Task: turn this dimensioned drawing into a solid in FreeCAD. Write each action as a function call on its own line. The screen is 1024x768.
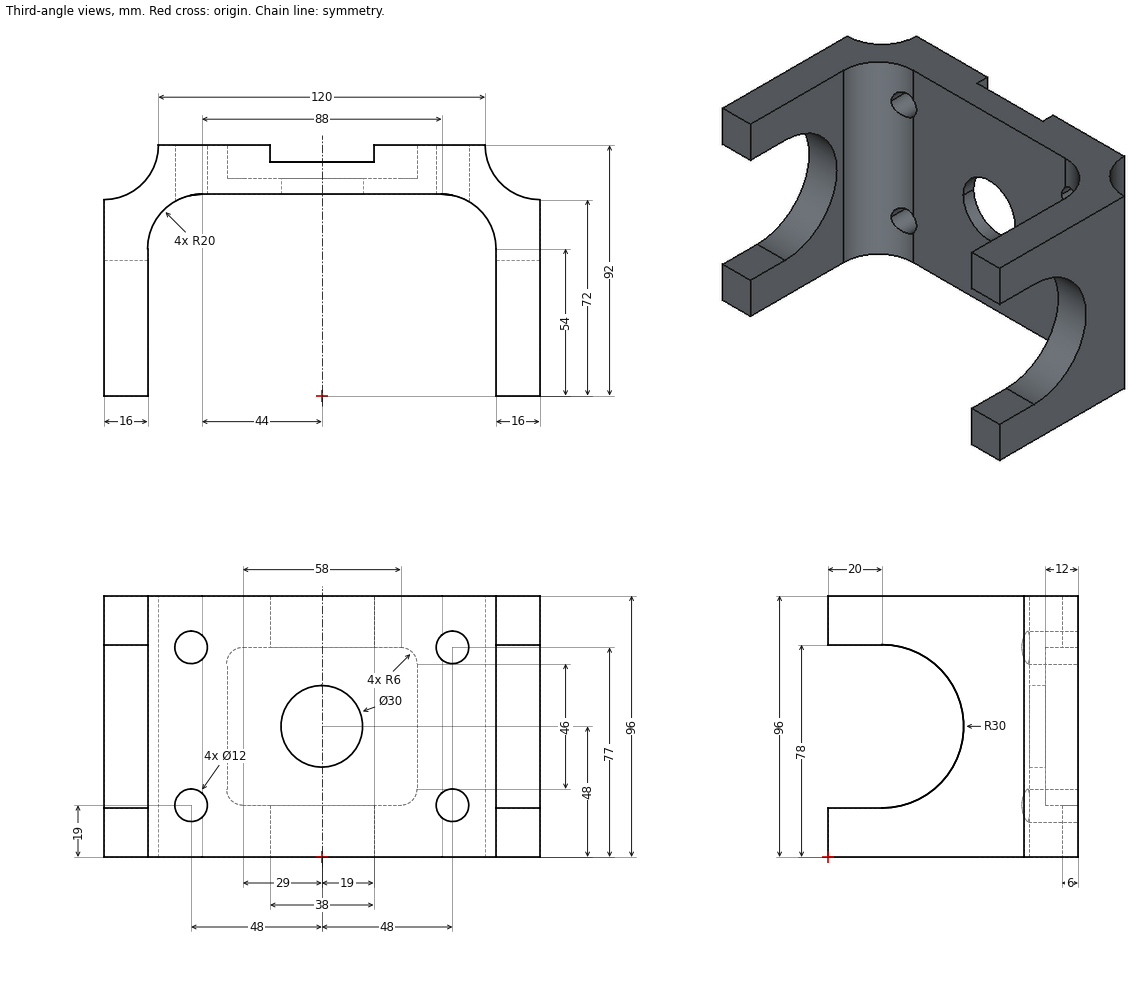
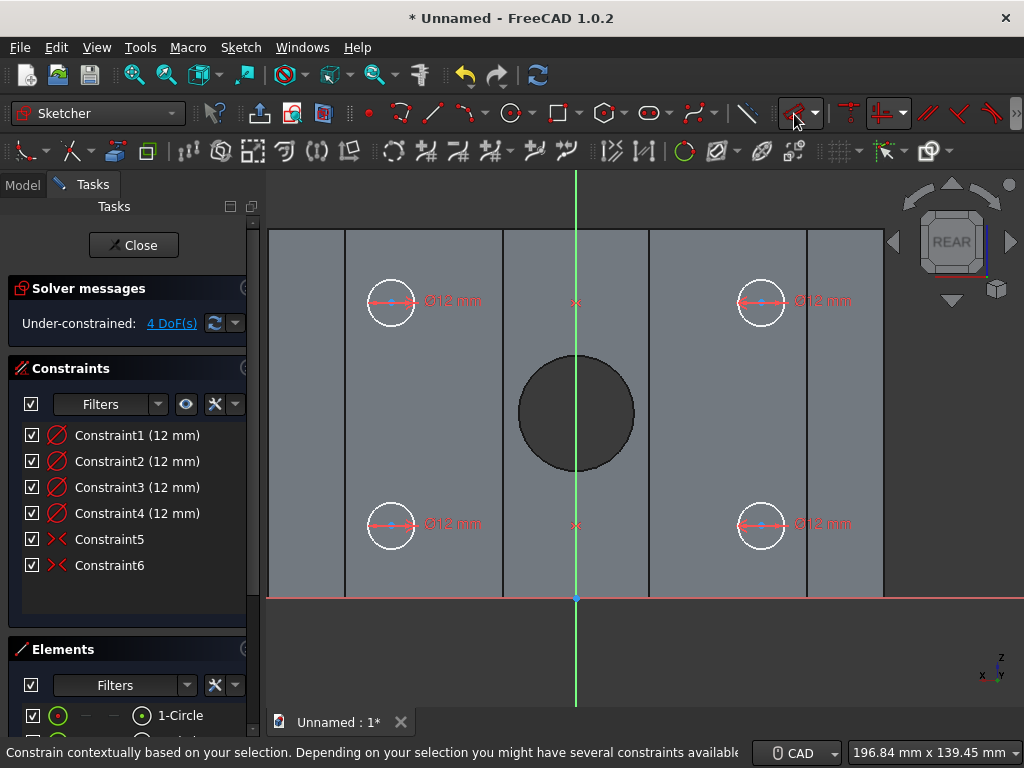
click(761, 526)
click(669, 632)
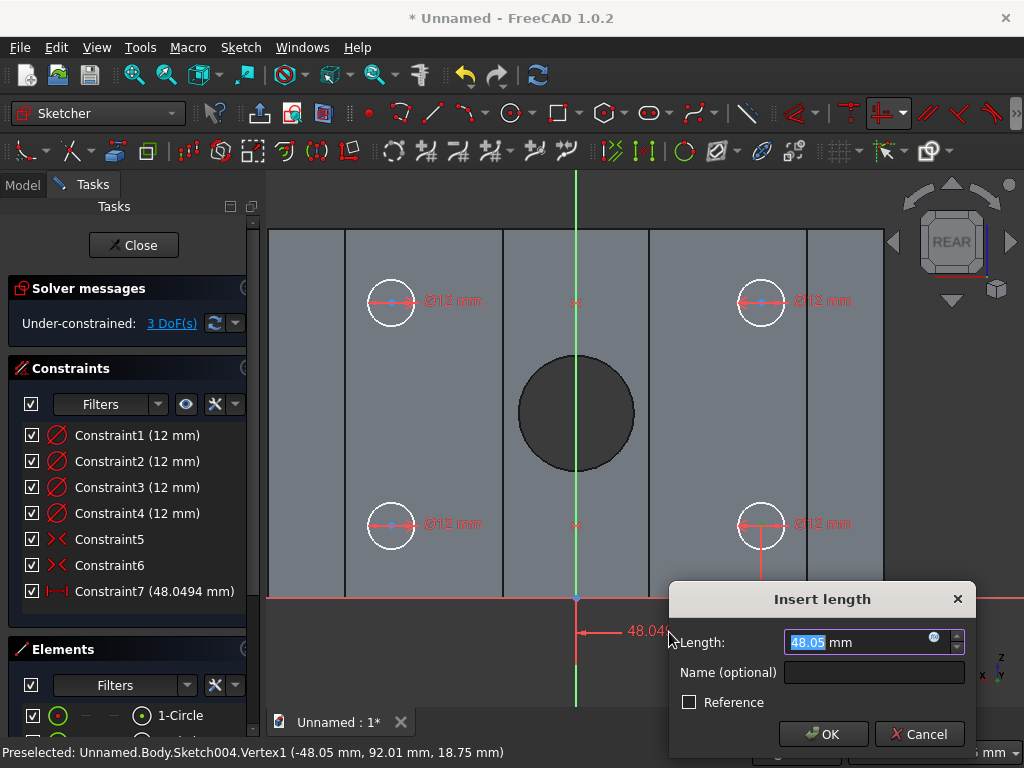
text(48)
key(Return)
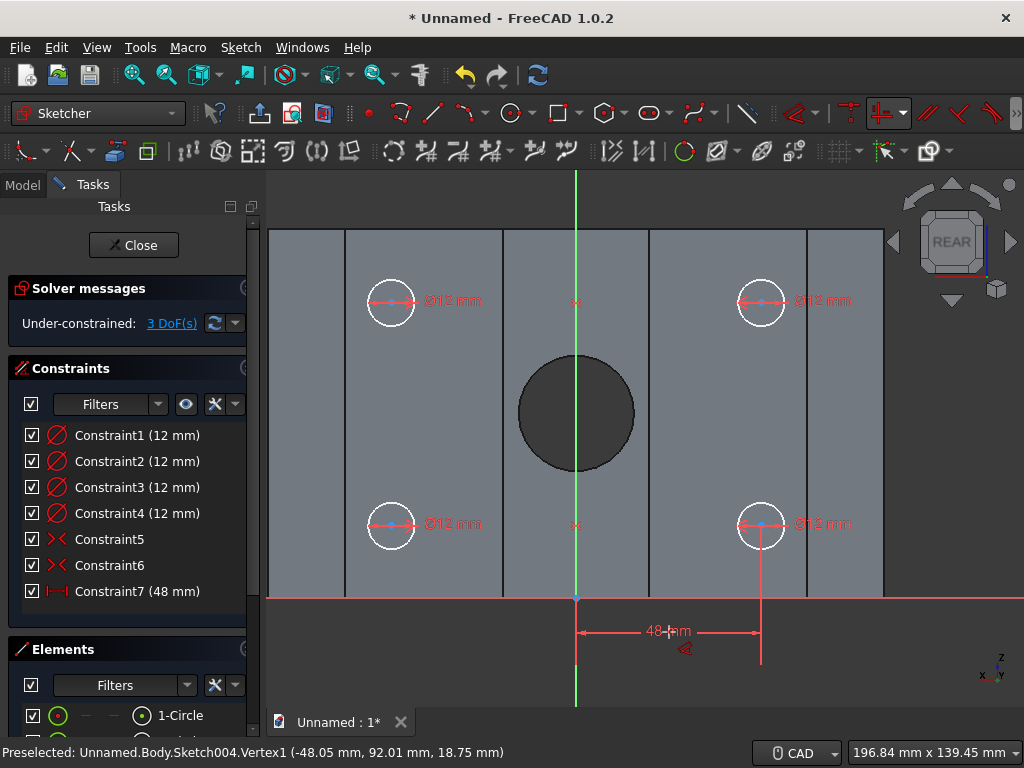
click(761, 526)
click(795, 562)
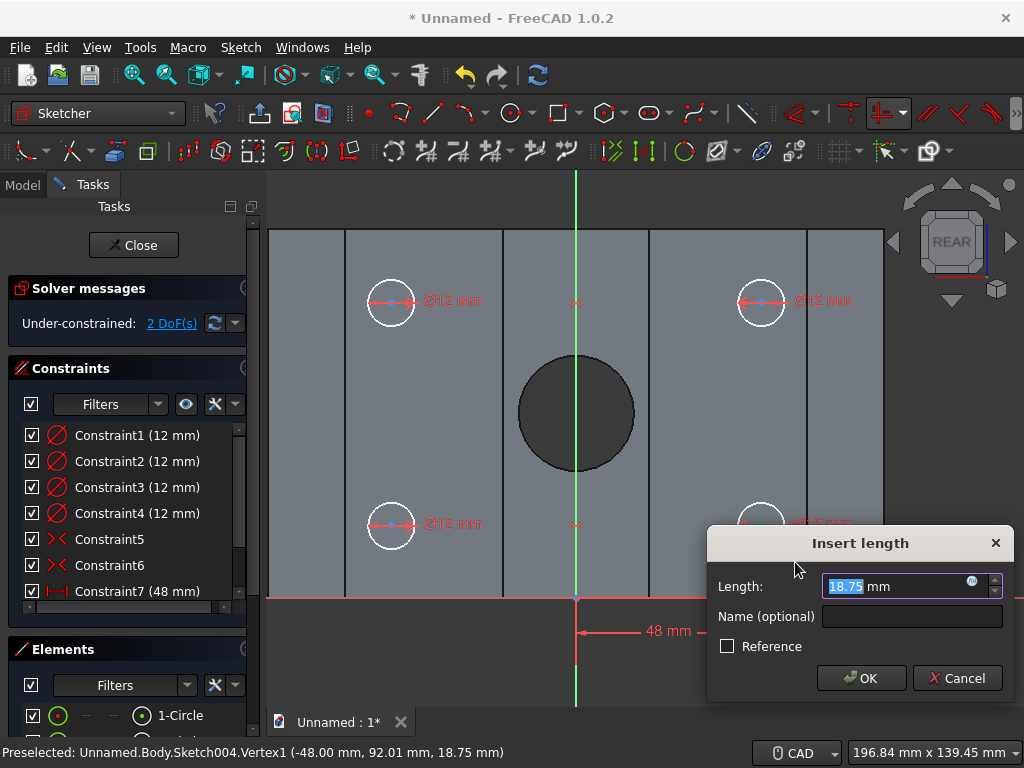
text(19)
key(Return)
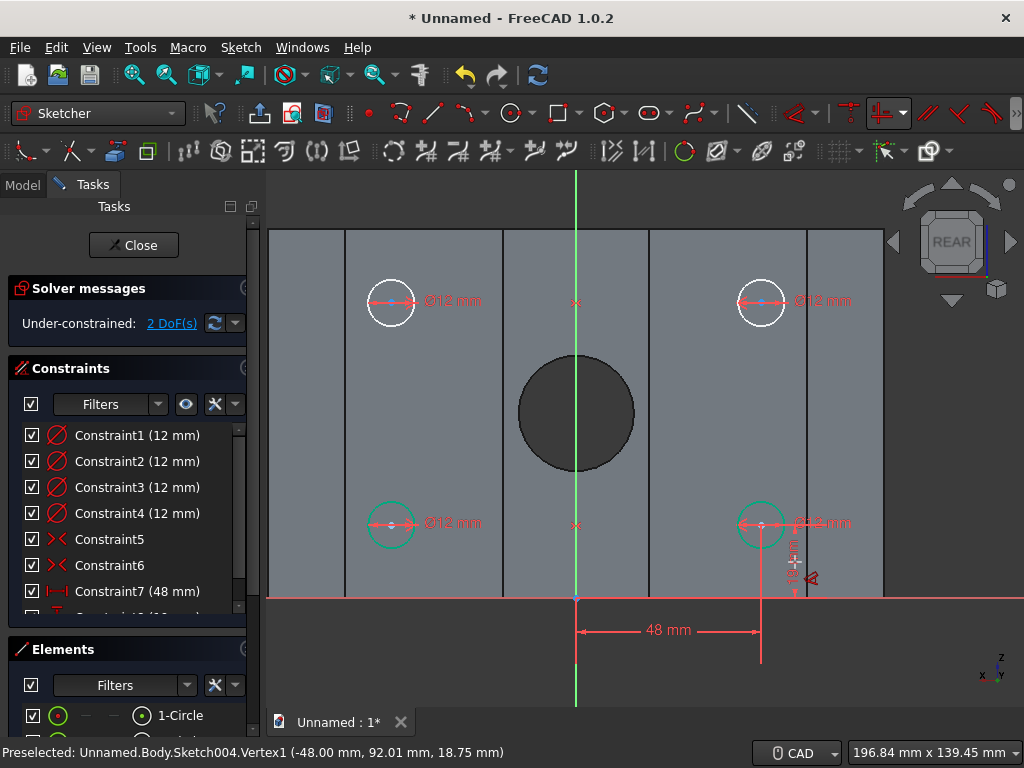
click(391, 303)
click(484, 632)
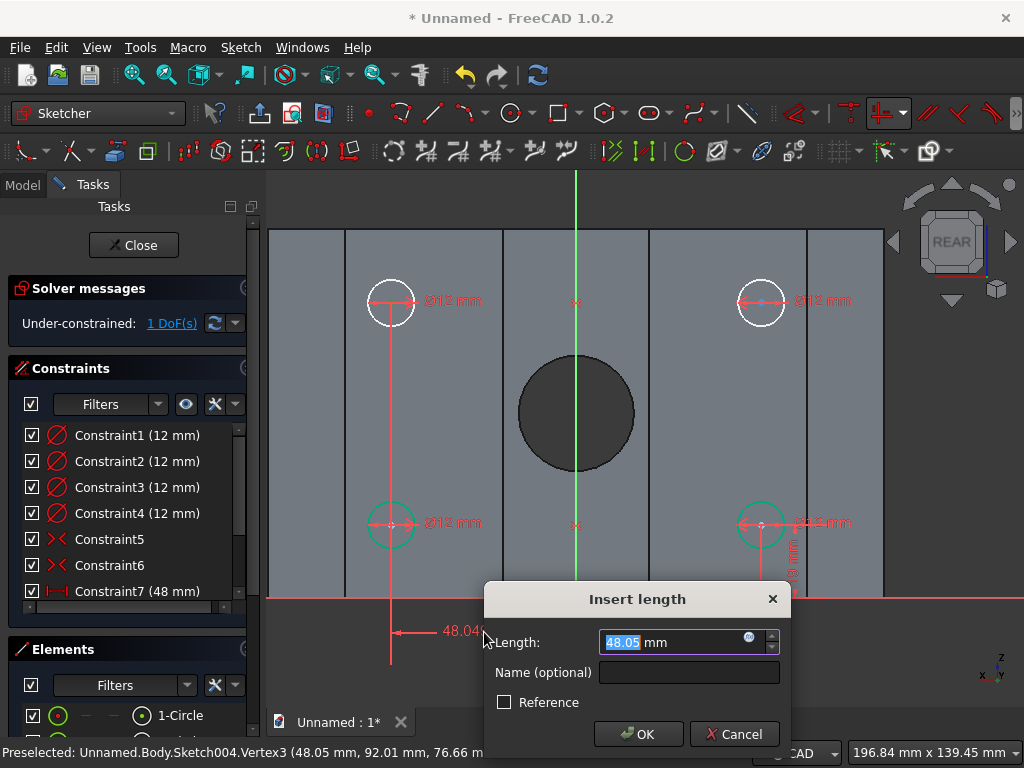
text(48)
key(Return)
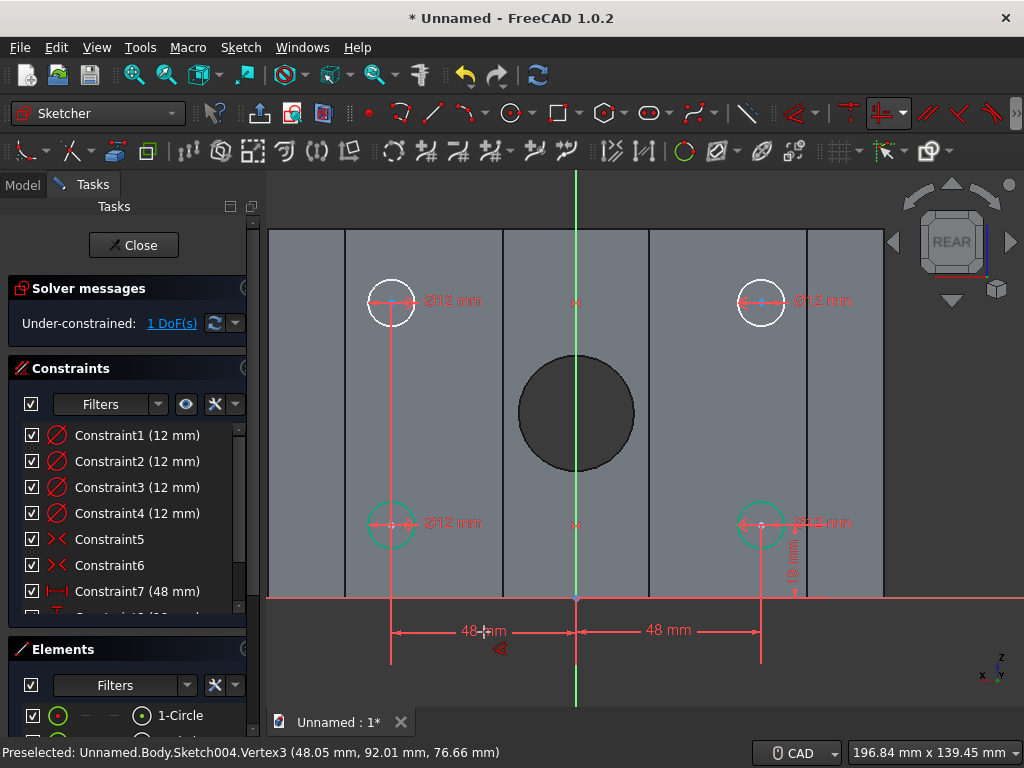
click(391, 303)
click(357, 451)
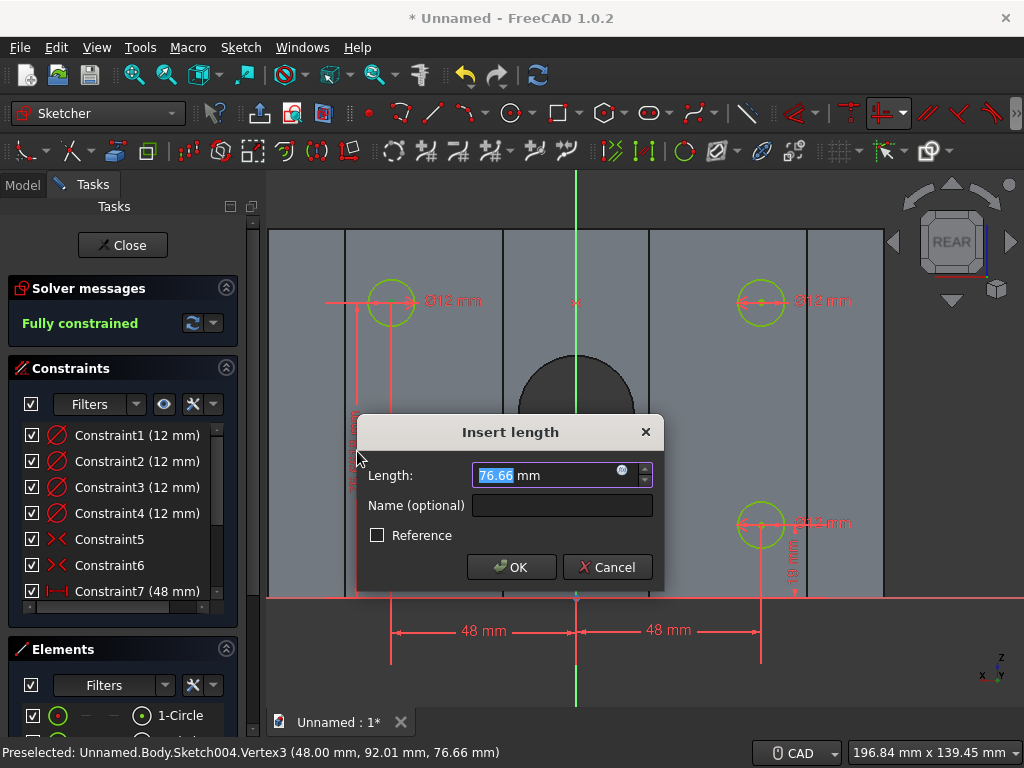
text(77)
key(Return)
key(Escape)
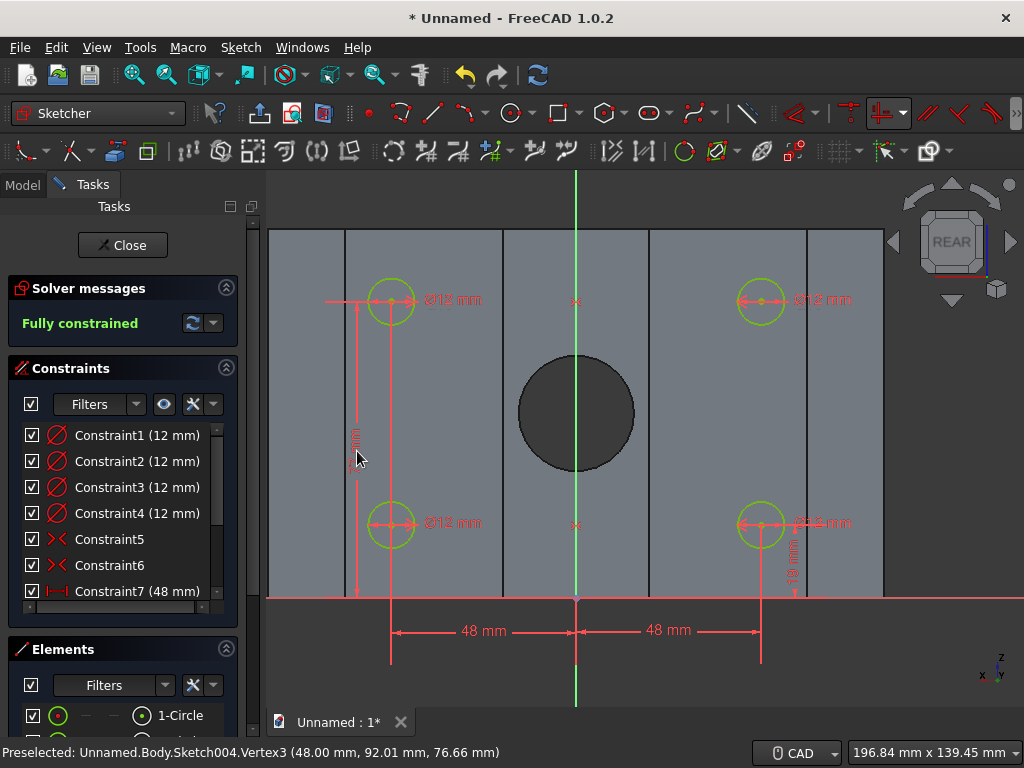
click(123, 245)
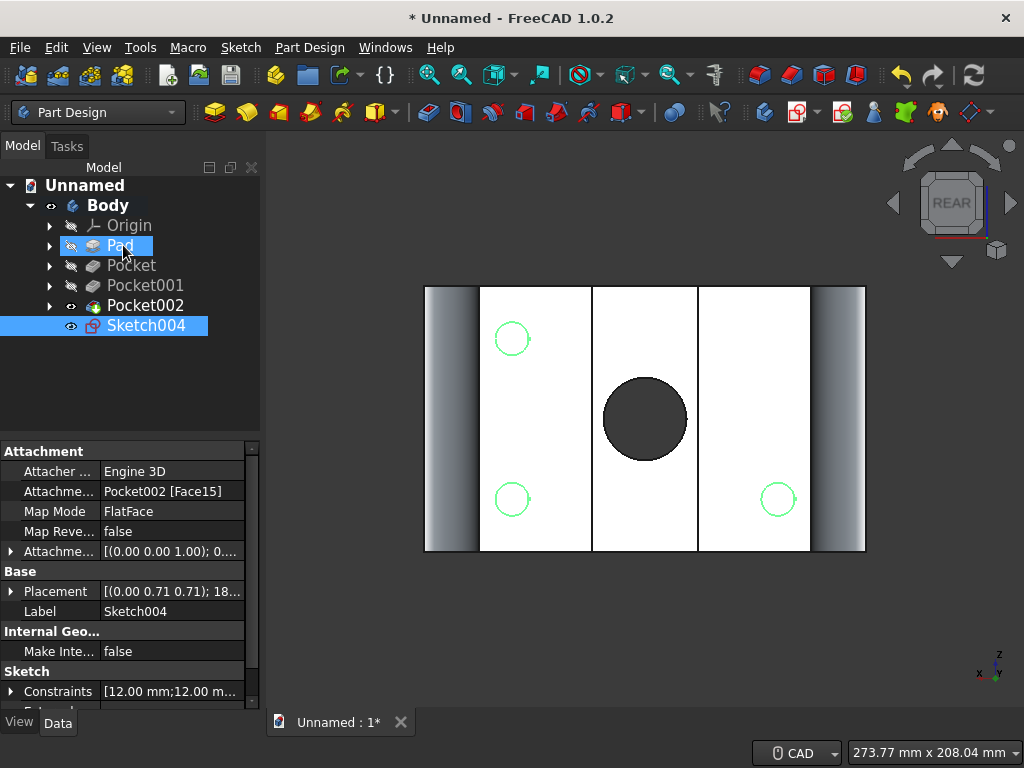
click(430, 112)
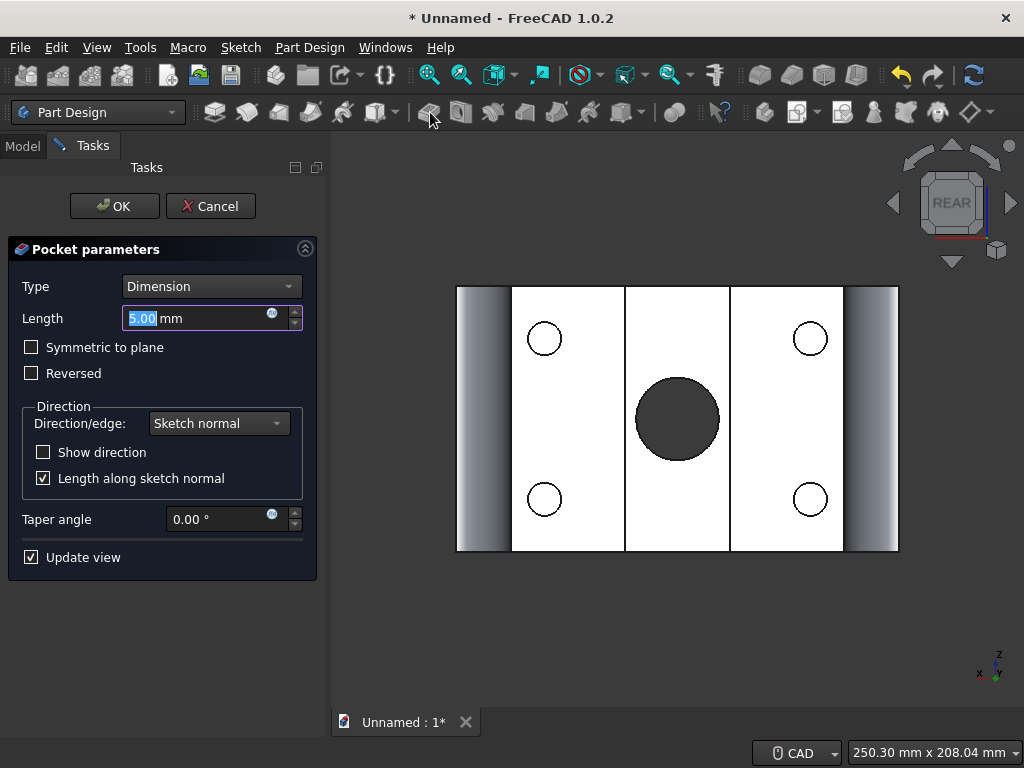
click(212, 286)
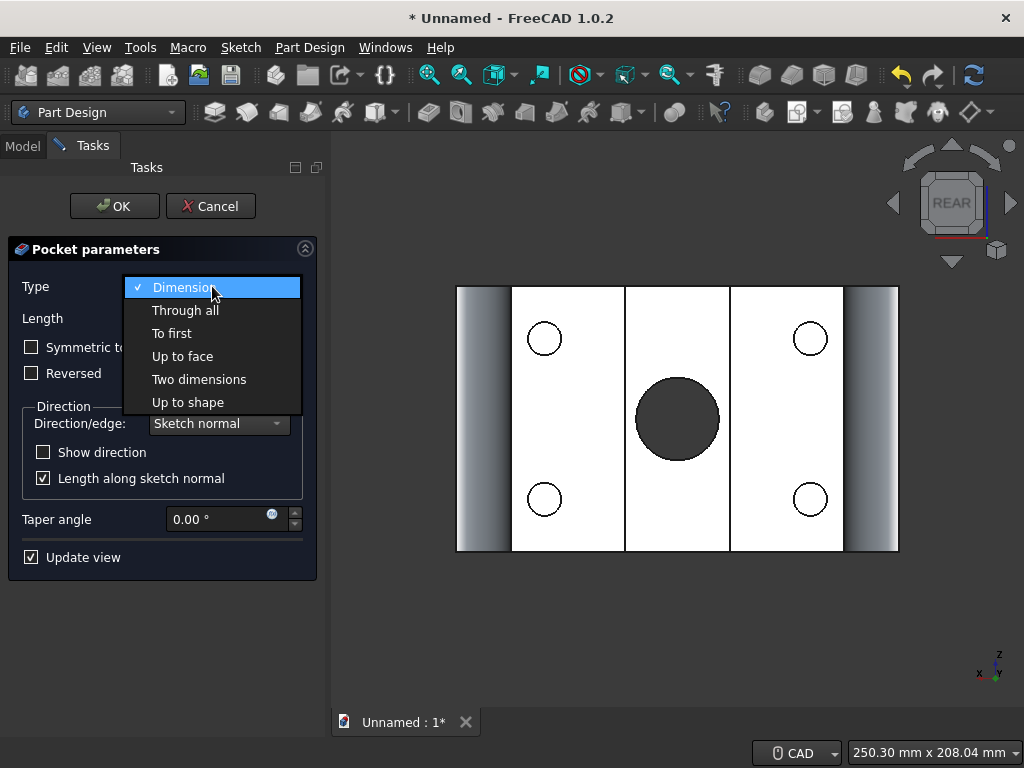
click(212, 310)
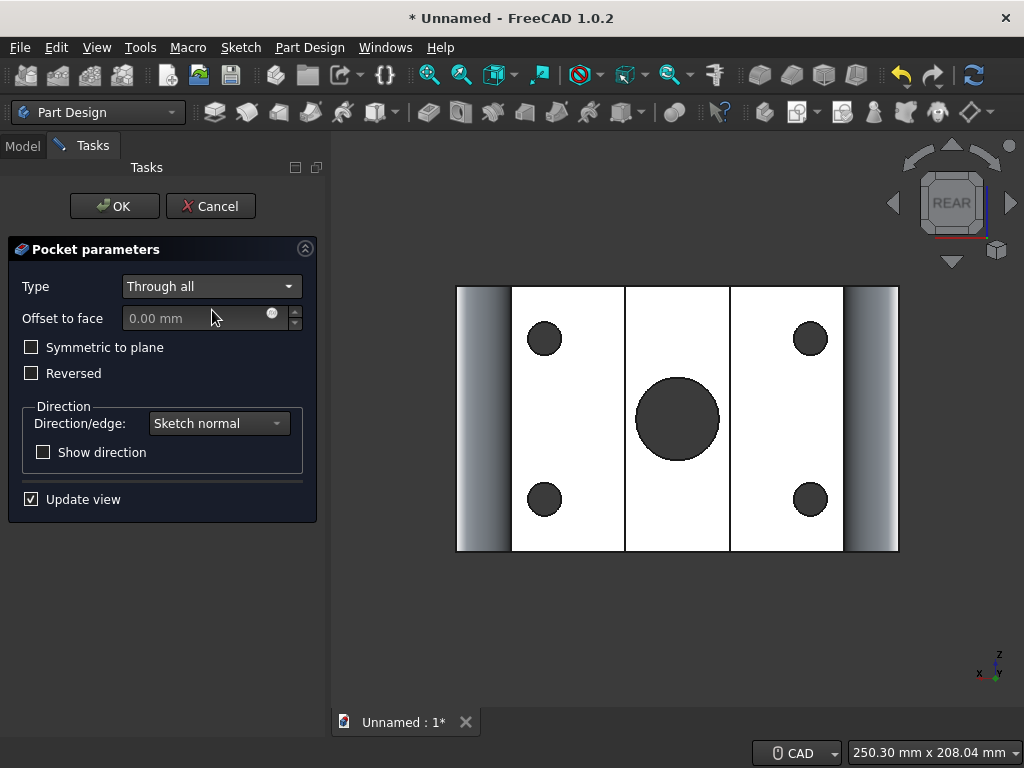
click(115, 206)